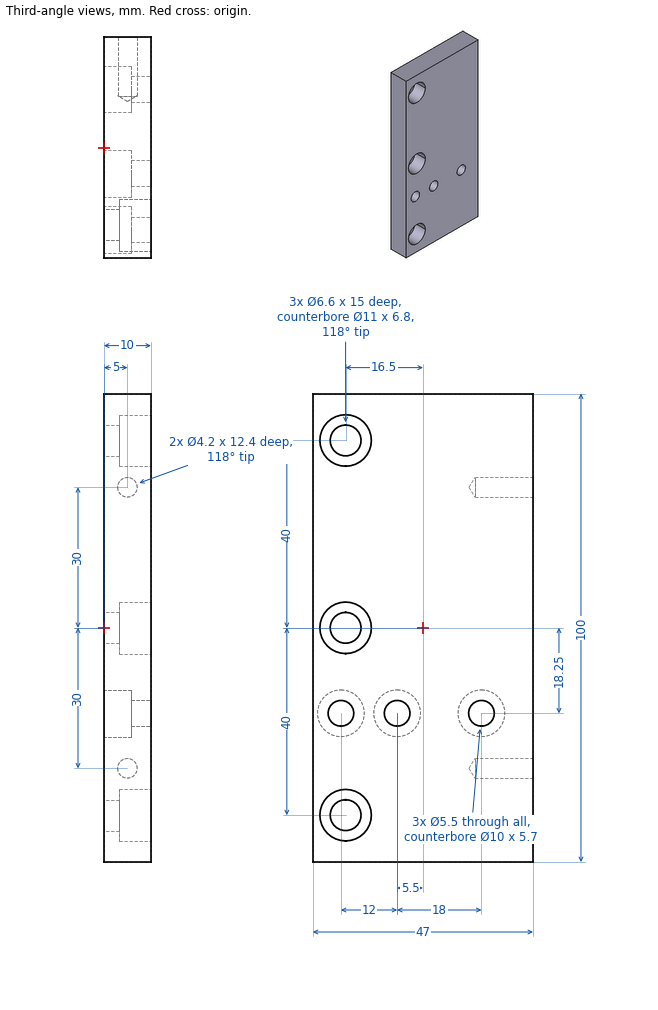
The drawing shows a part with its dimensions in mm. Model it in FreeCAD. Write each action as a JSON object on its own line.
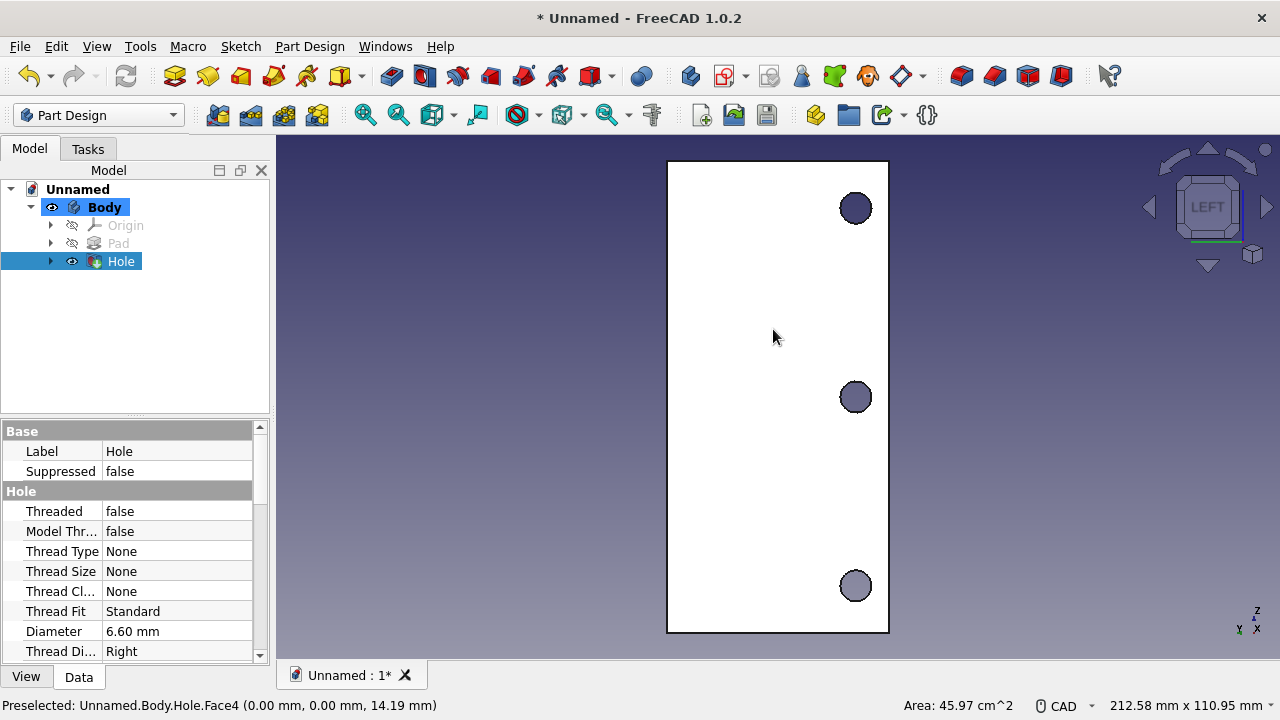
{"action": "left_click", "coordinate": [724, 76]}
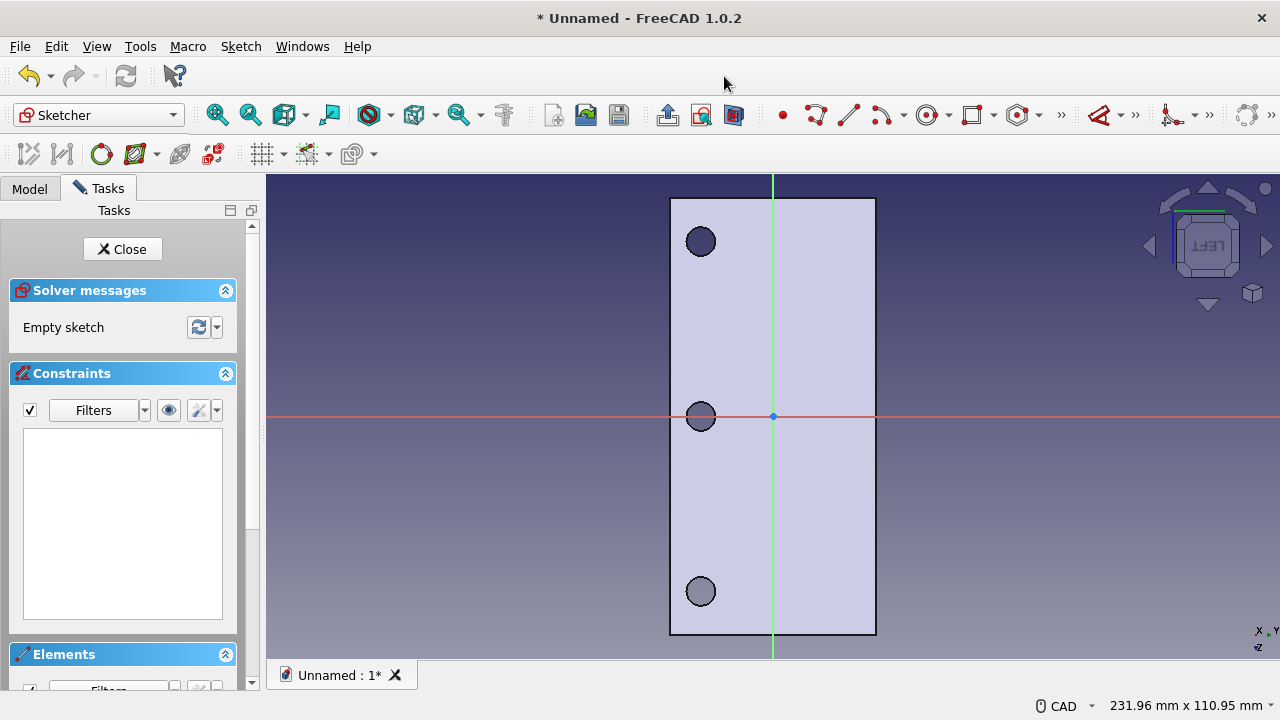
{"action": "scroll", "coordinate": [787, 351], "scroll_direction": "up", "scroll_amount": 6}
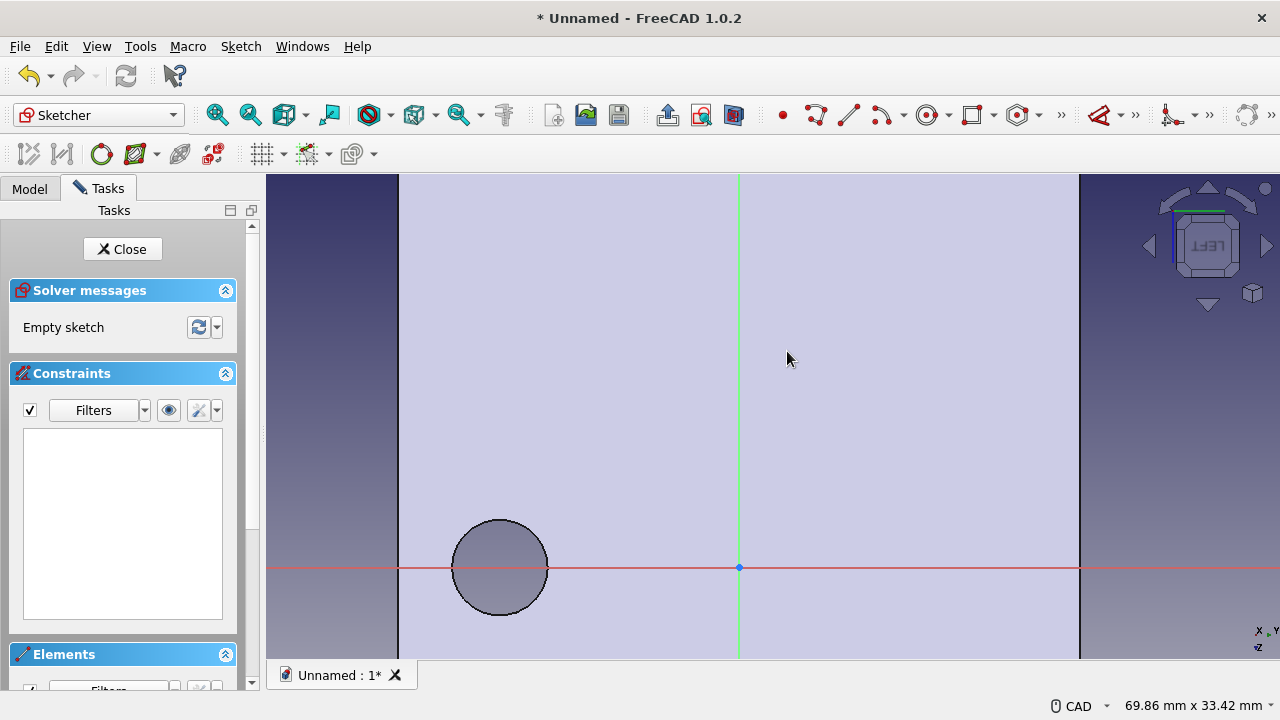
{"action": "left_click", "coordinate": [926, 116]}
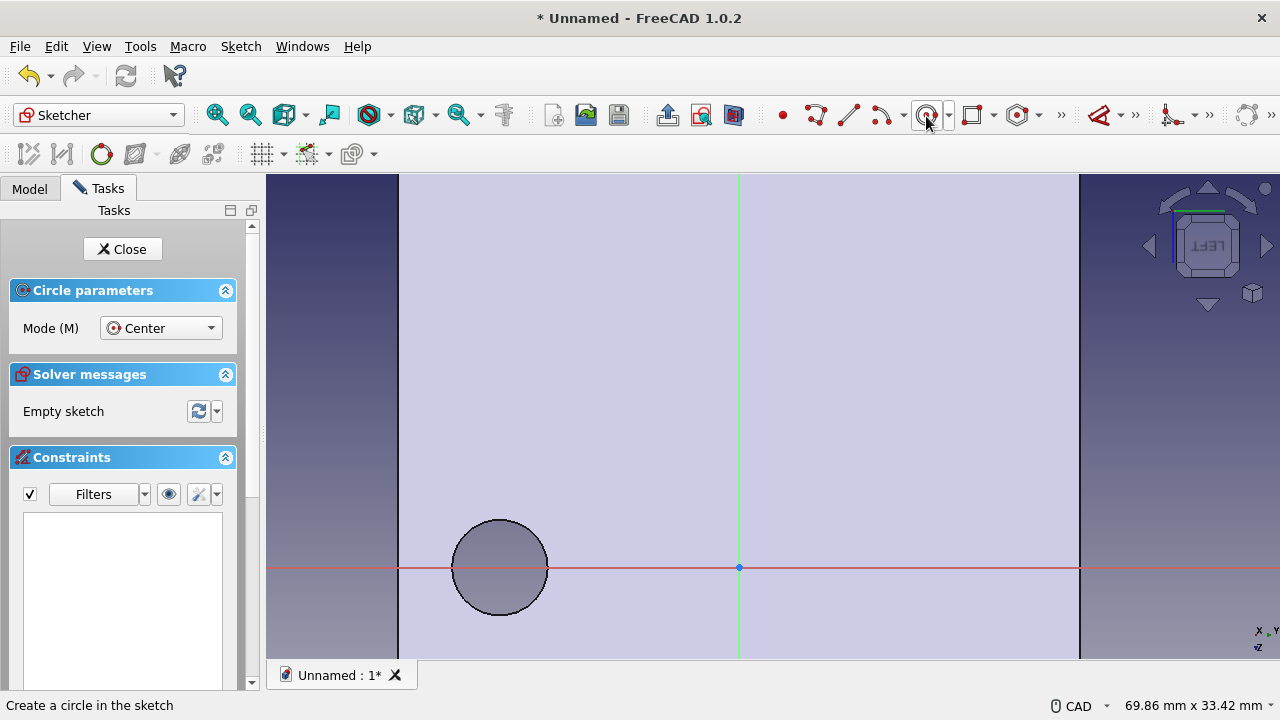
{"action": "left_click", "coordinate": [921, 303]}
{"action": "mouse_move", "coordinate": [949, 275]}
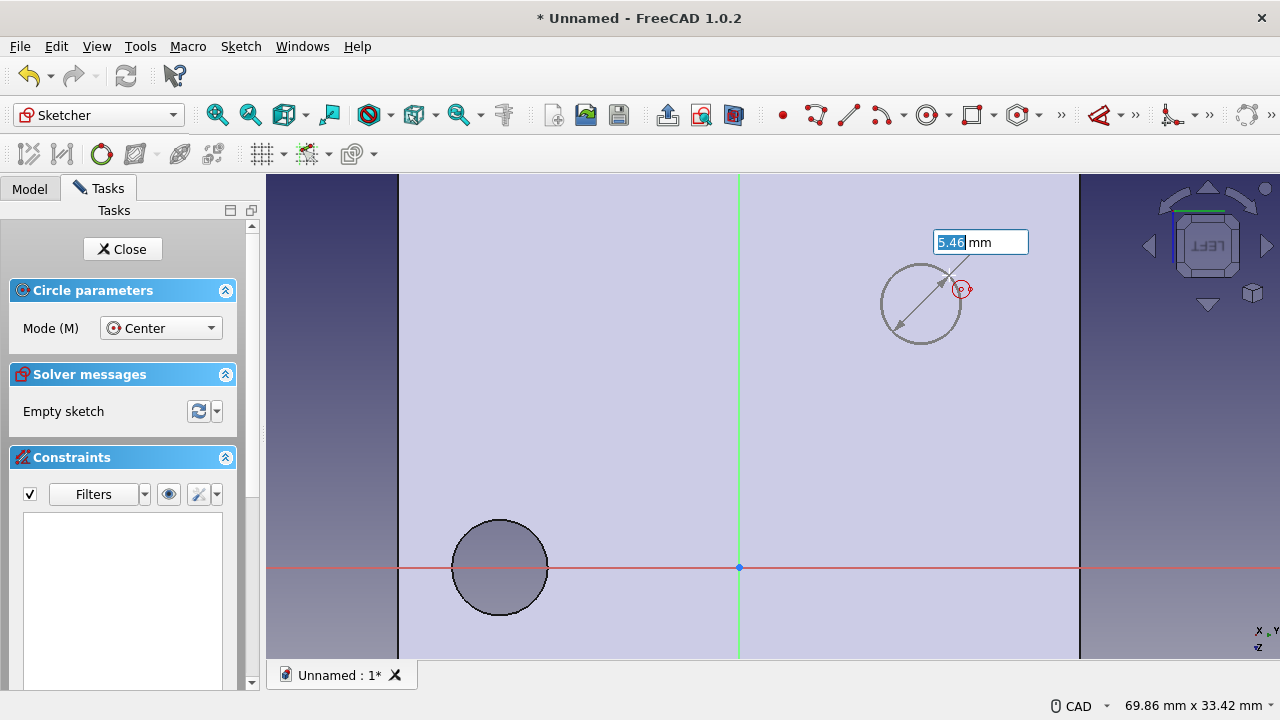
{"action": "type", "text": "5.5"}
{"action": "key", "text": "Return"}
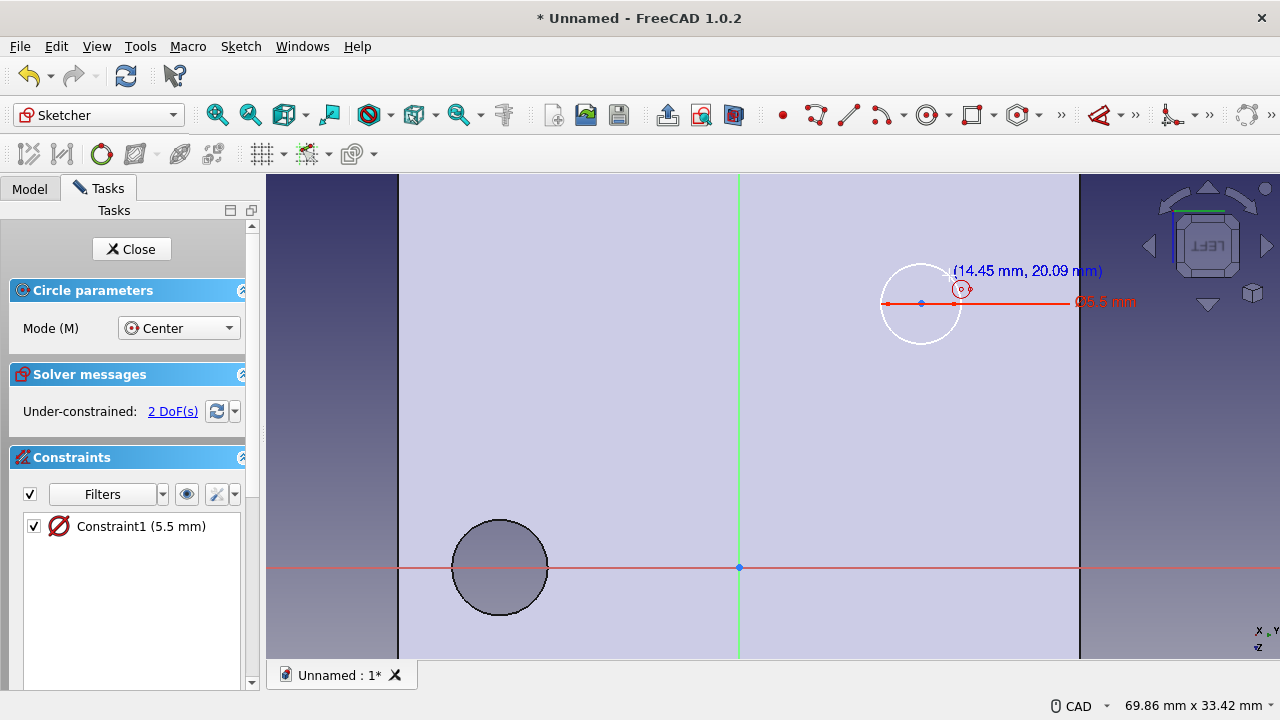
{"action": "left_click", "coordinate": [659, 303]}
{"action": "mouse_move", "coordinate": [688, 275]}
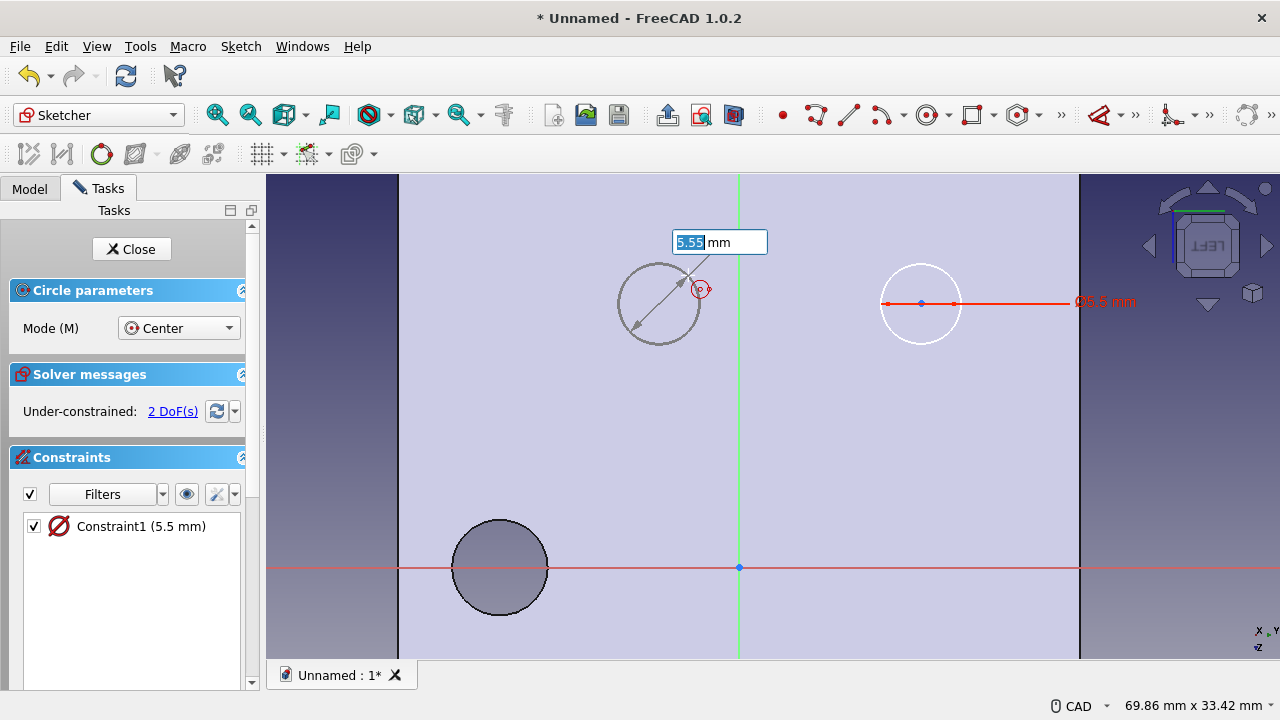
{"action": "type", "text": "5.5"}
{"action": "key", "text": "Return"}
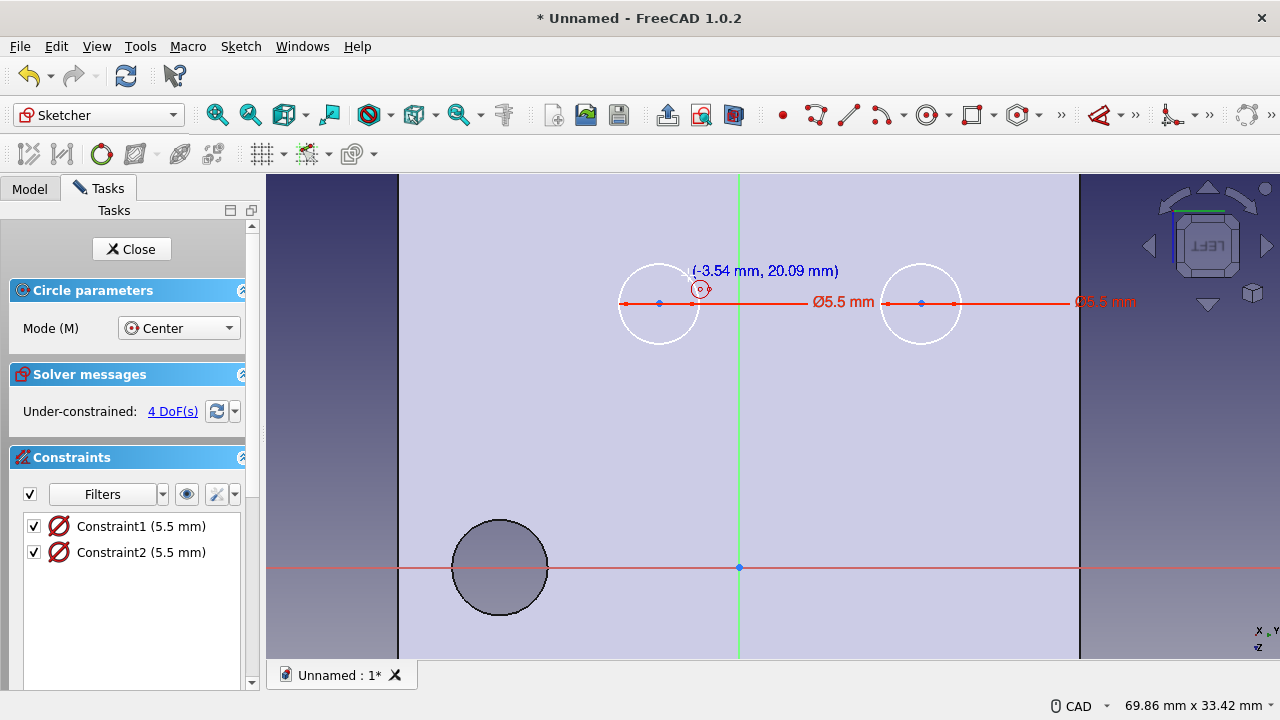
{"action": "left_click", "coordinate": [485, 303]}
{"action": "mouse_move", "coordinate": [514, 275]}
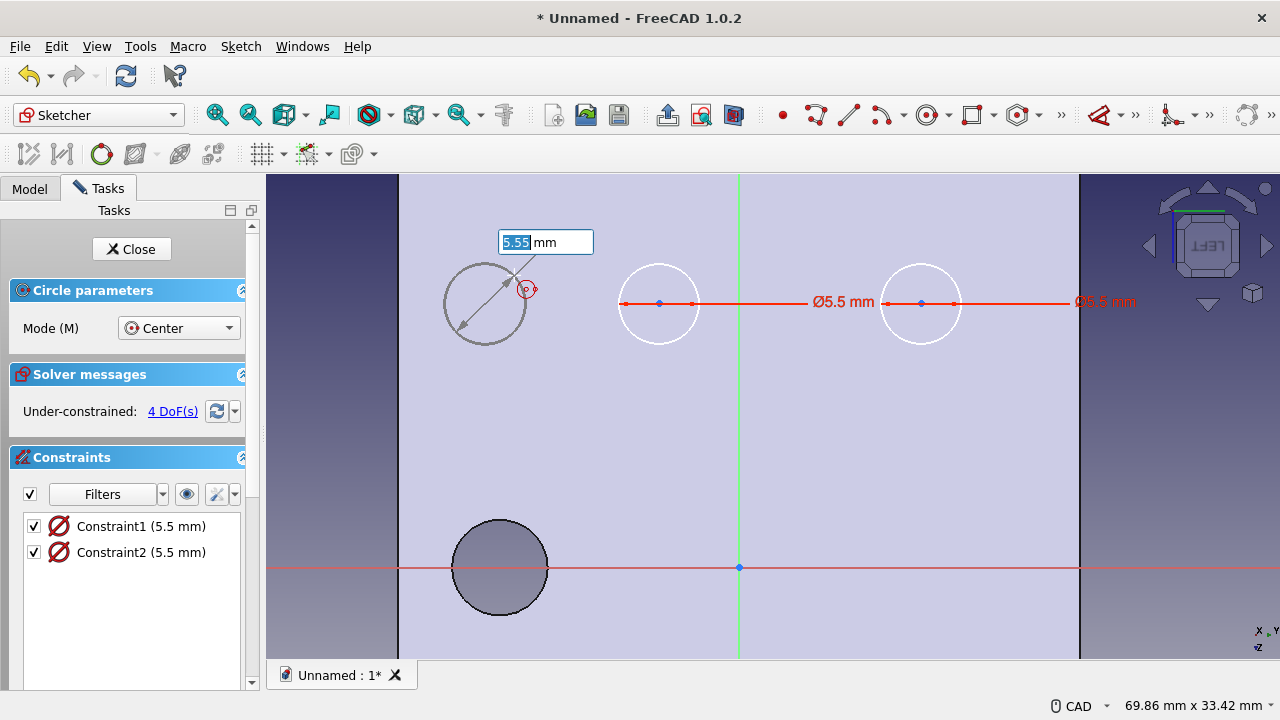
{"action": "type", "text": "5.5"}
{"action": "key", "text": "Return"}
{"action": "key", "text": "Escape"}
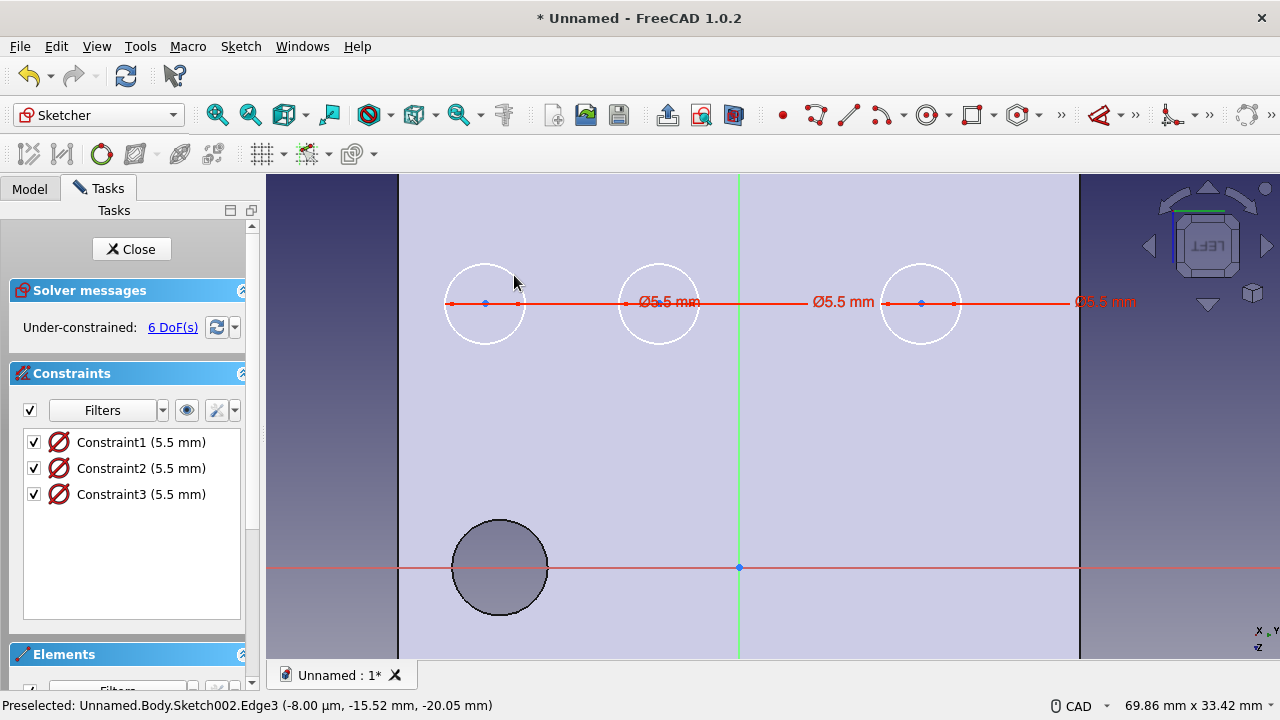
{"action": "left_click", "coordinate": [921, 304]}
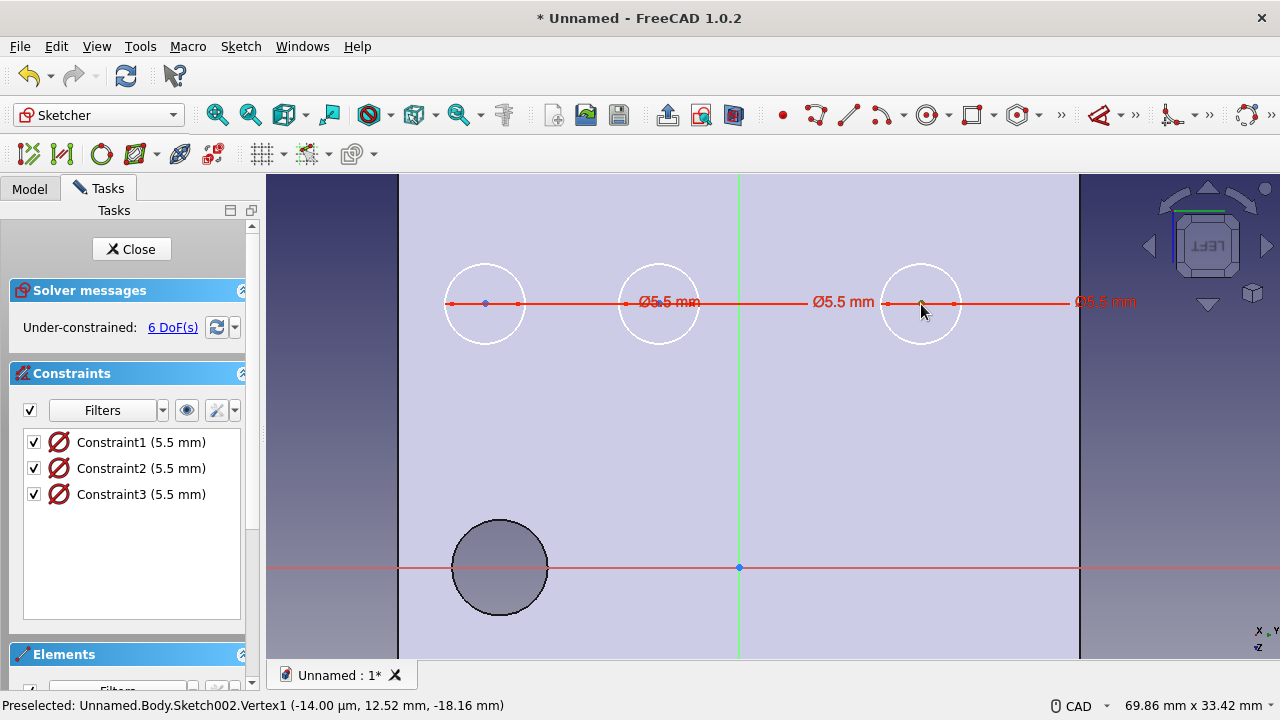
{"action": "left_click", "coordinate": [659, 304]}